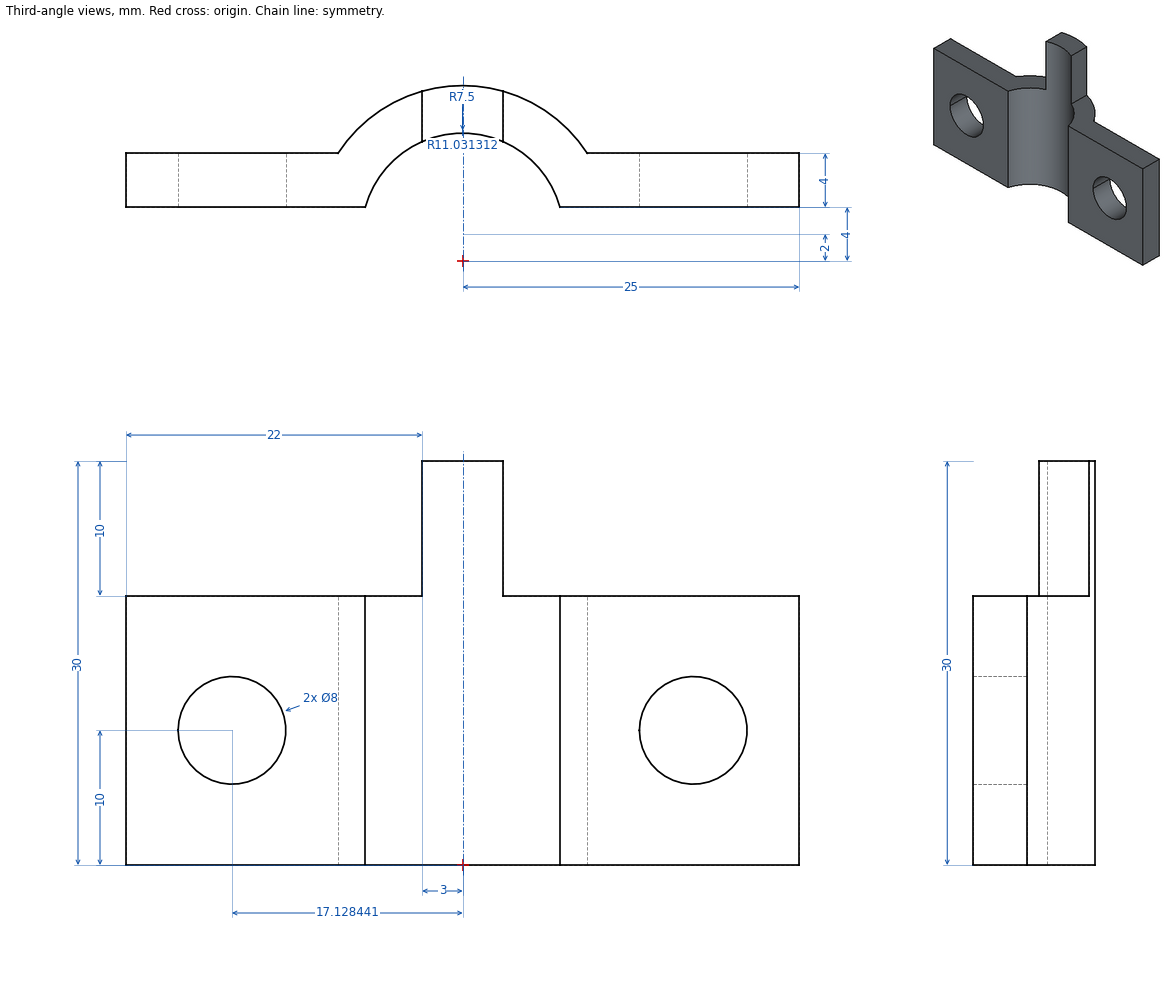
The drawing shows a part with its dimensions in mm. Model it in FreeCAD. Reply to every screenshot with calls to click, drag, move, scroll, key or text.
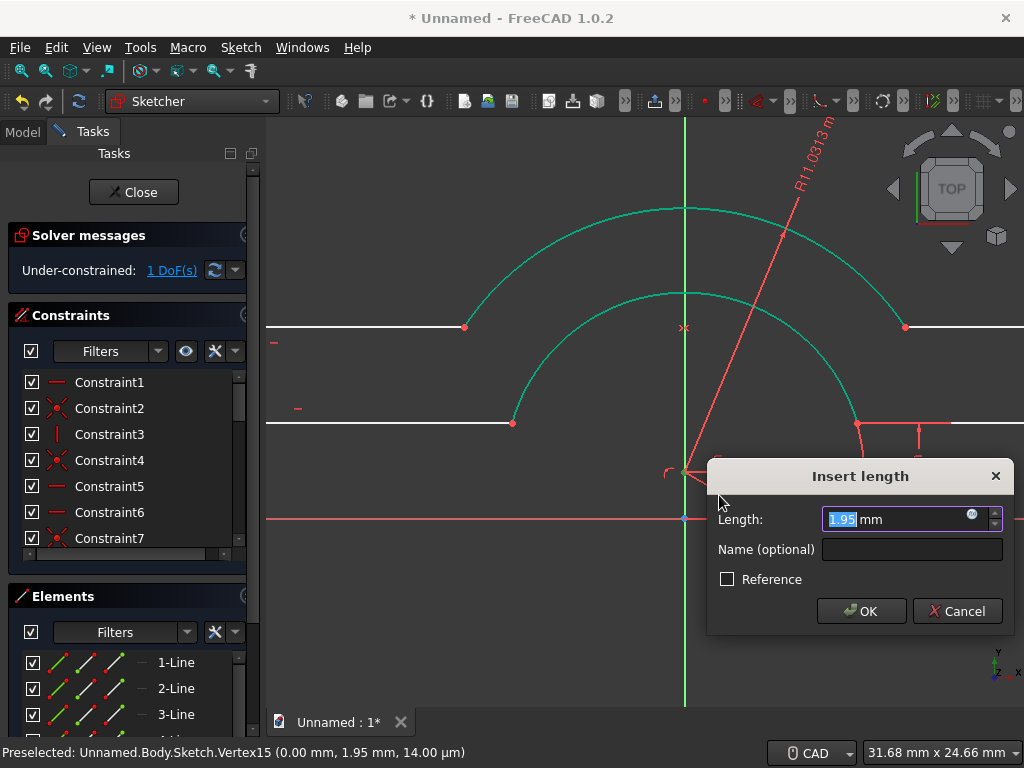
text(2)
key(Return)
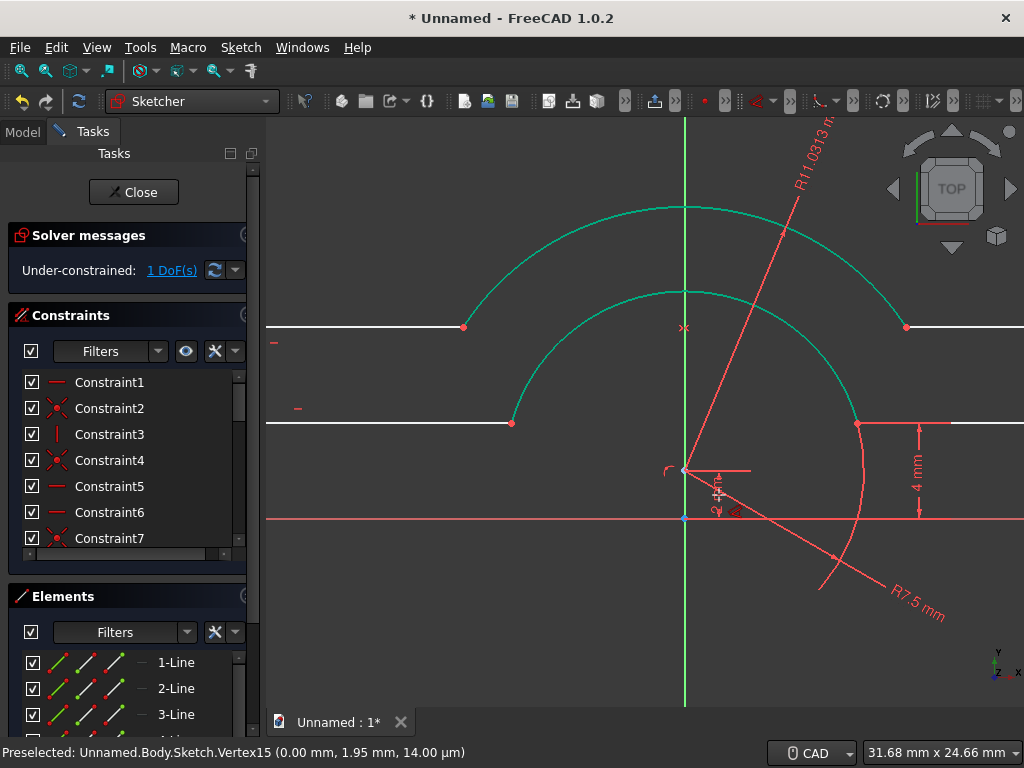
scroll(514, 441, down, 5)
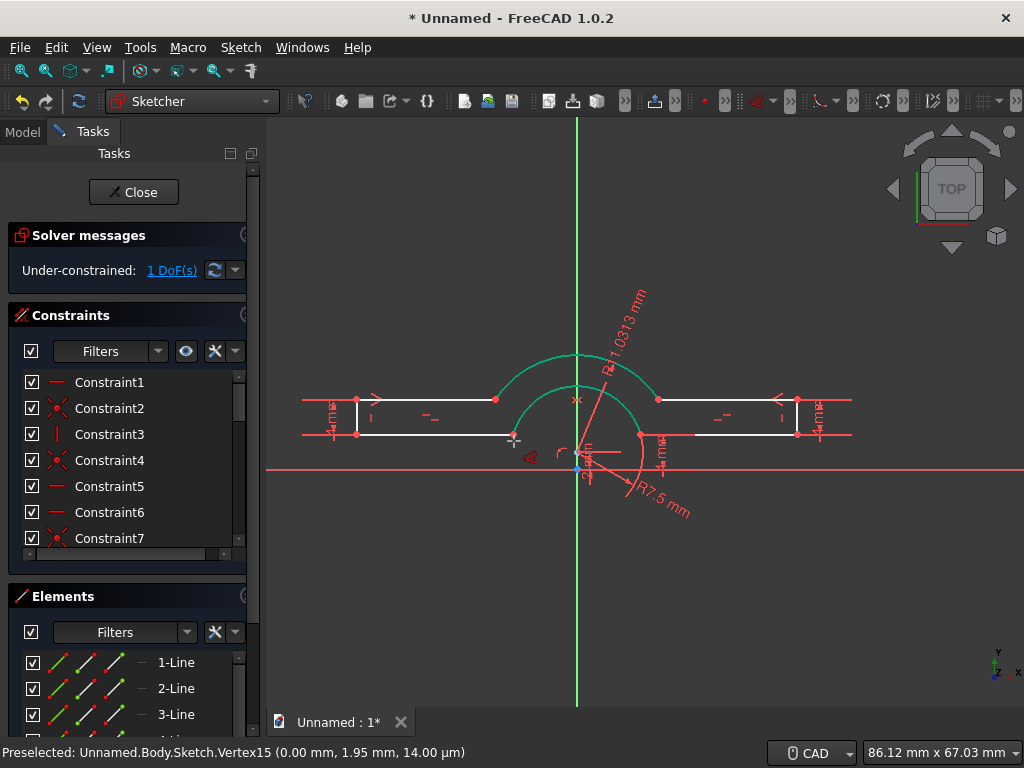
click(797, 435)
click(738, 504)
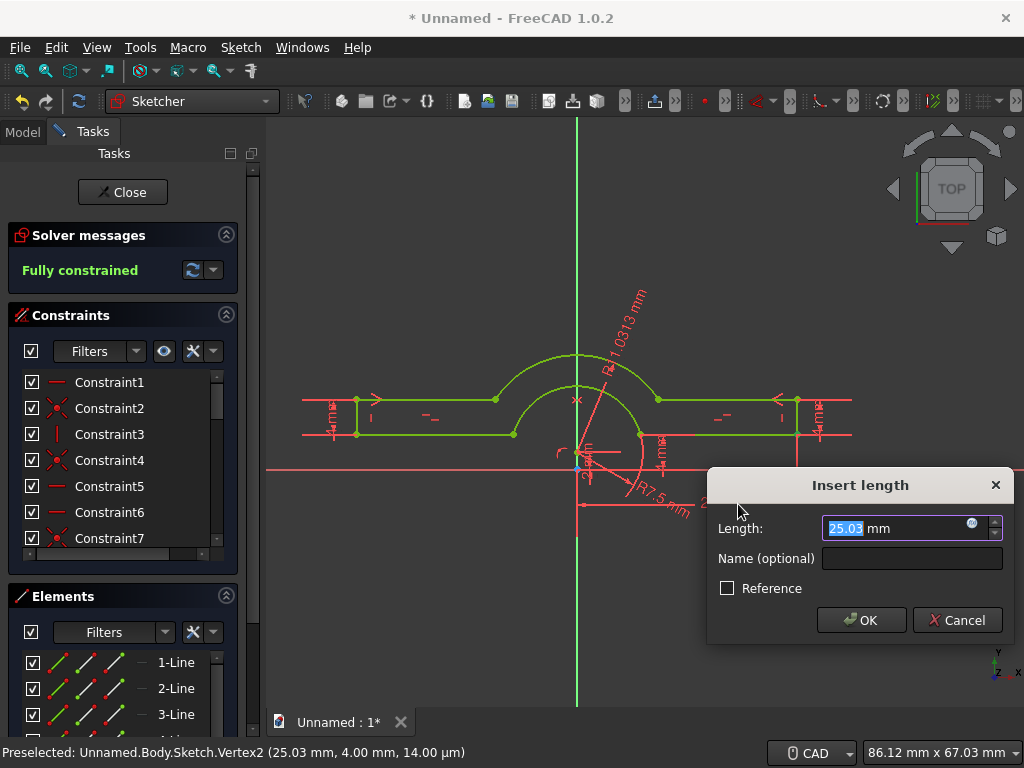
text(25)
key(Return)
key(Escape)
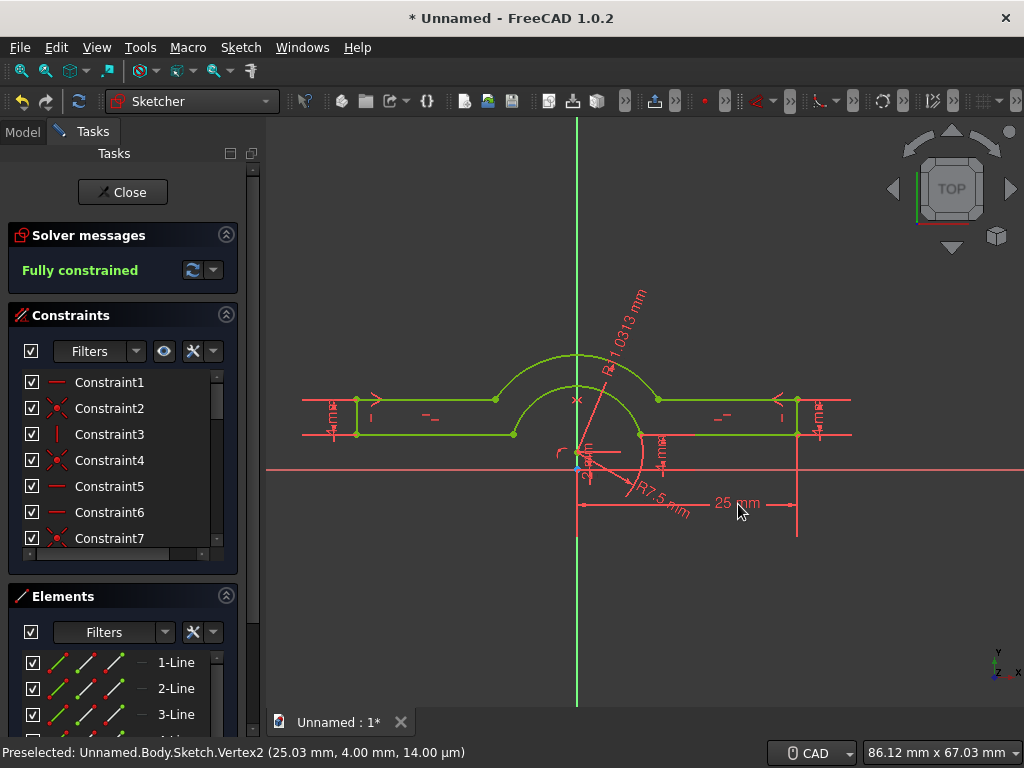
click(123, 192)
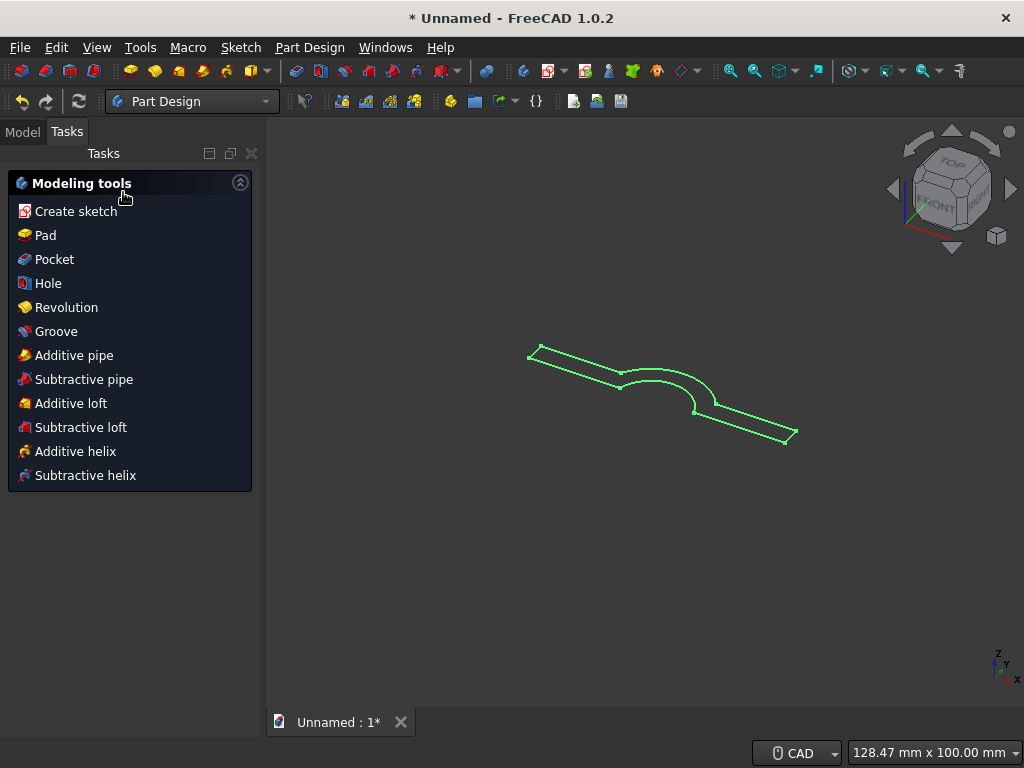
click(132, 72)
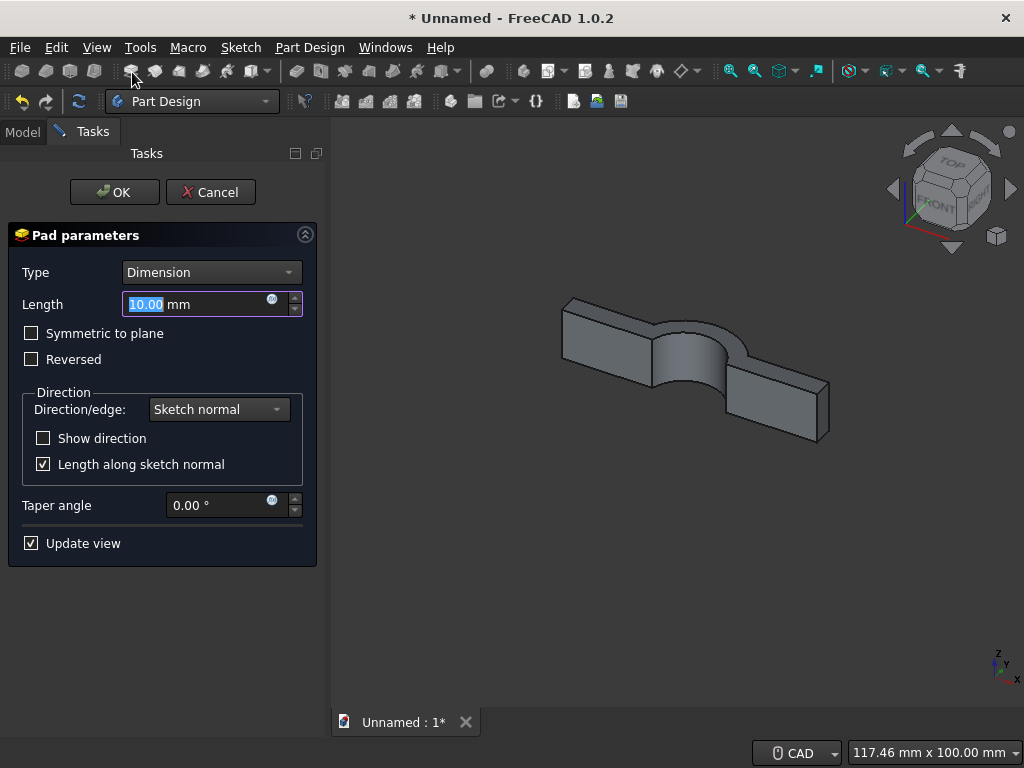
text(30)
key(Tab)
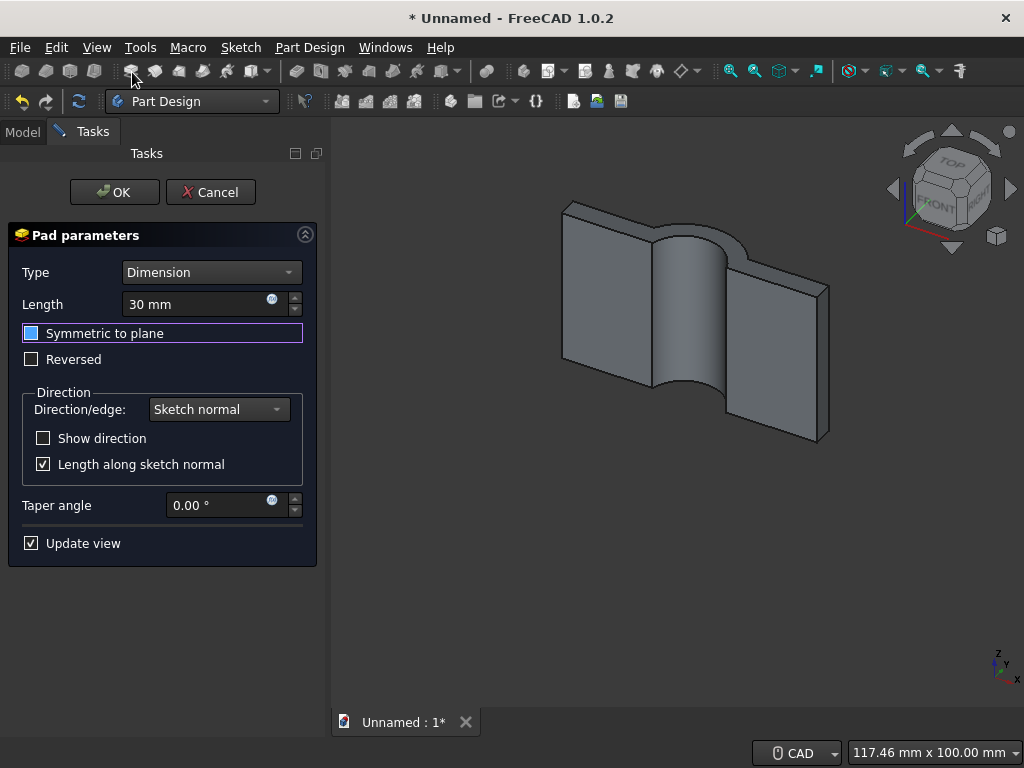
click(115, 192)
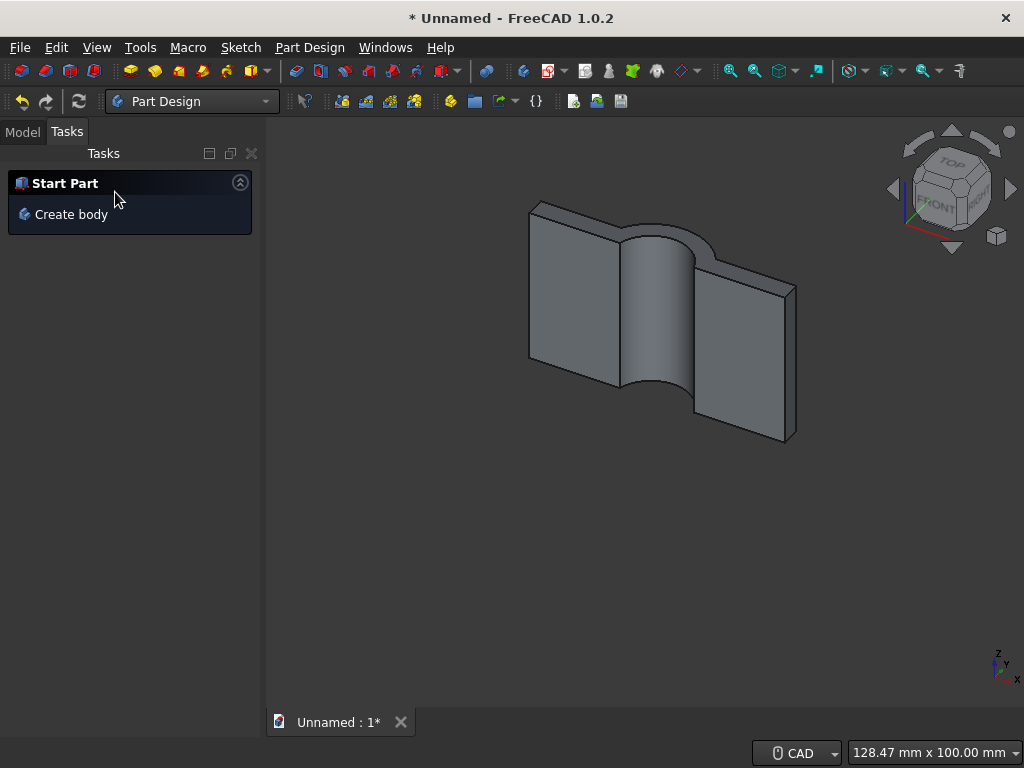
click(732, 72)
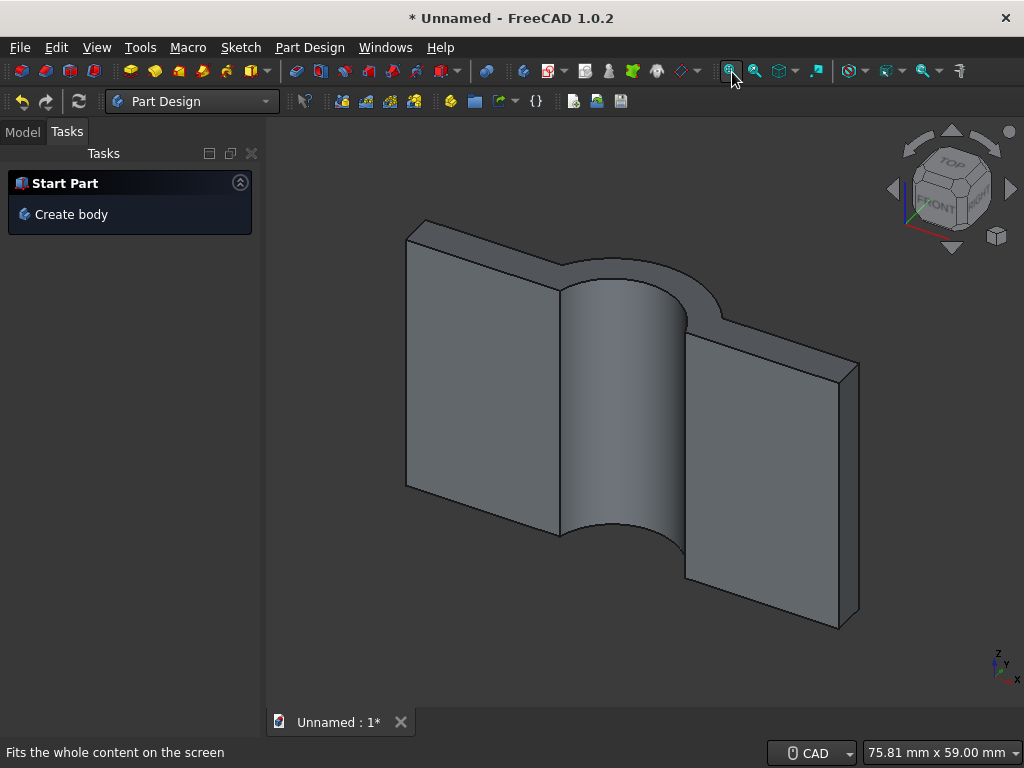
click(483, 352)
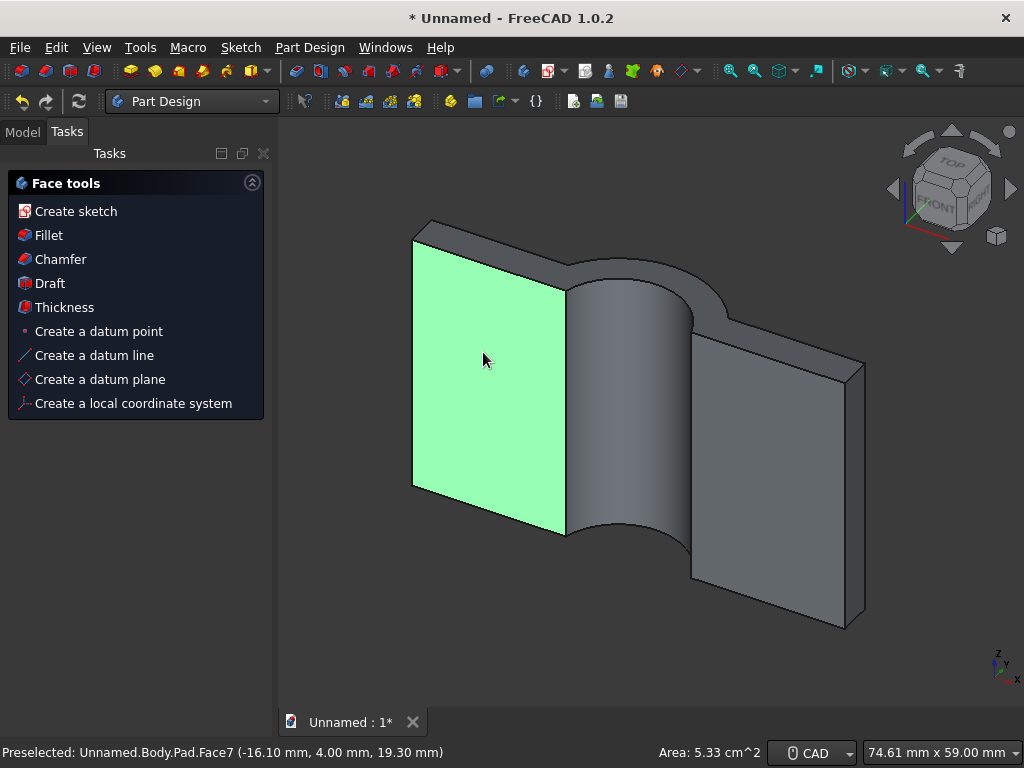
click(548, 72)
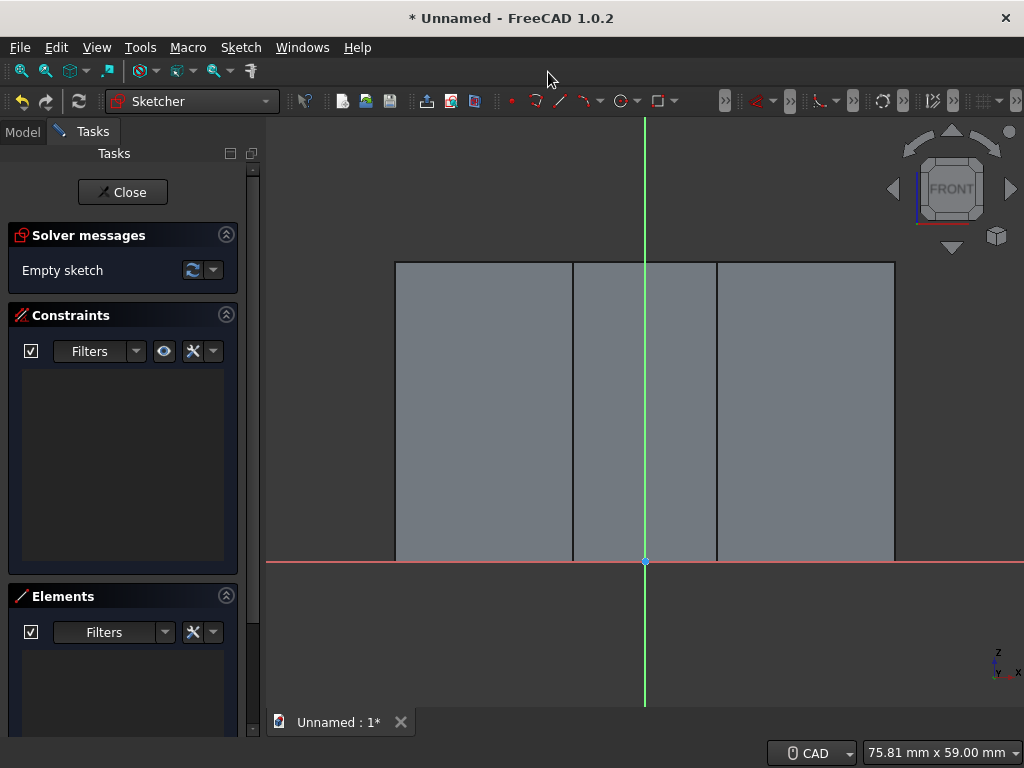
scroll(294, 412, down, 1)